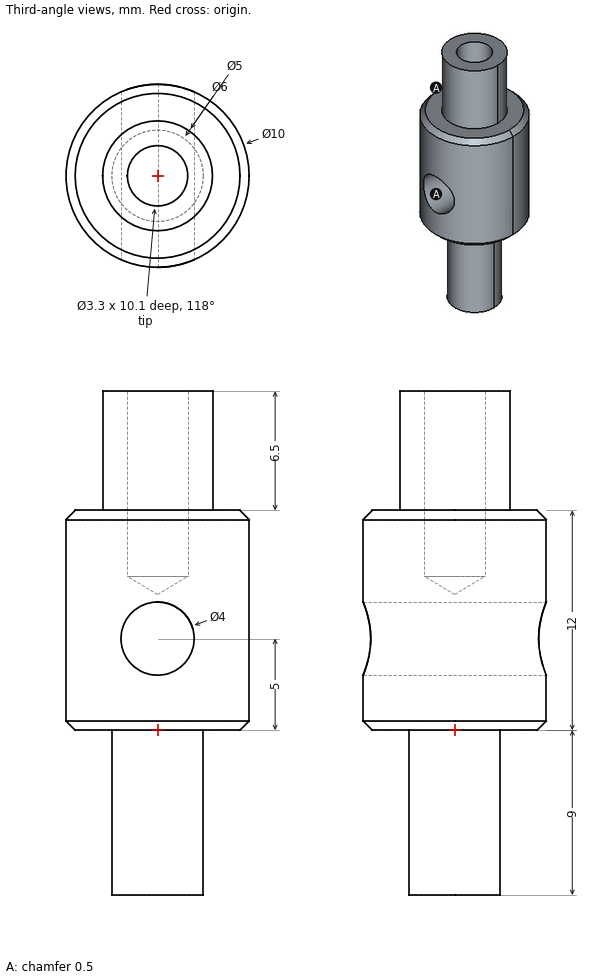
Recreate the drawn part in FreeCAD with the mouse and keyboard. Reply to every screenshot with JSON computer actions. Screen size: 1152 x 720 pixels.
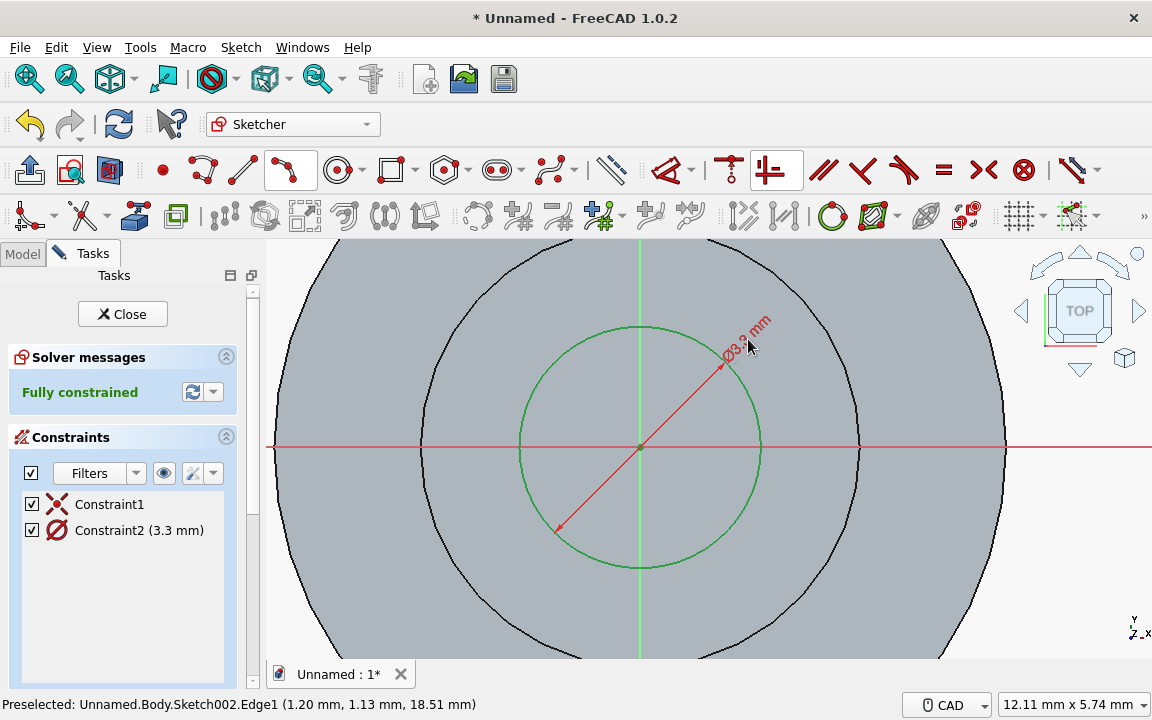
{"action": "left_click", "coordinate": [123, 314]}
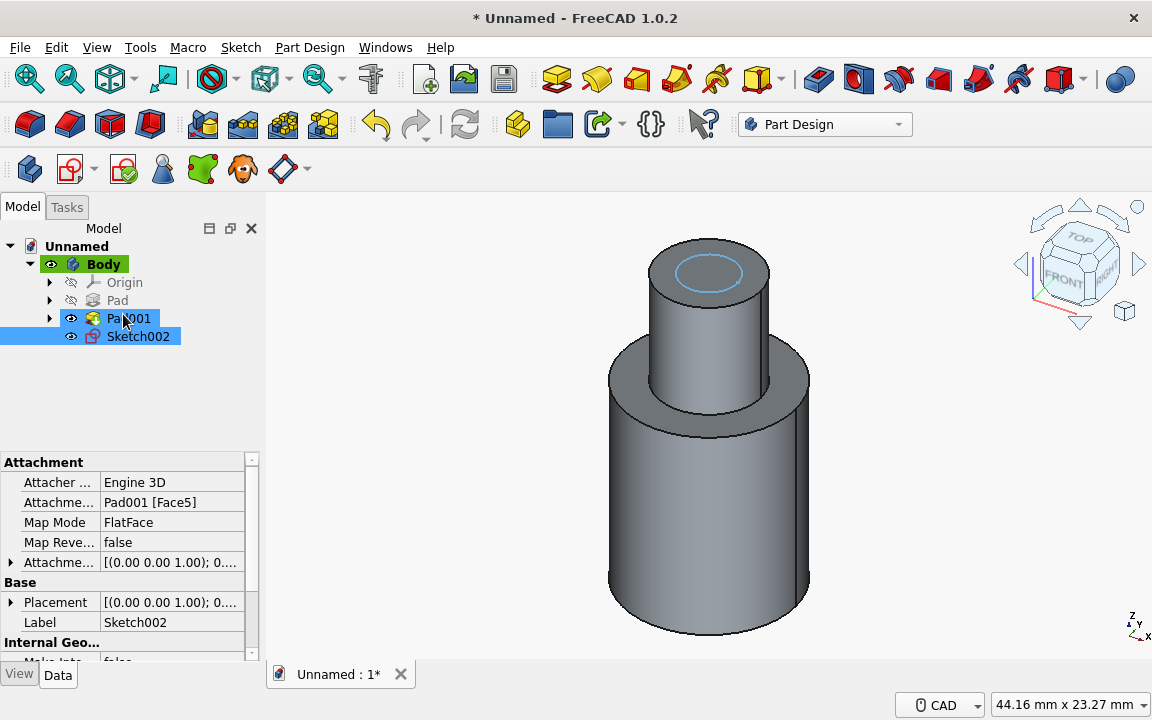
{"action": "left_click", "coordinate": [860, 80]}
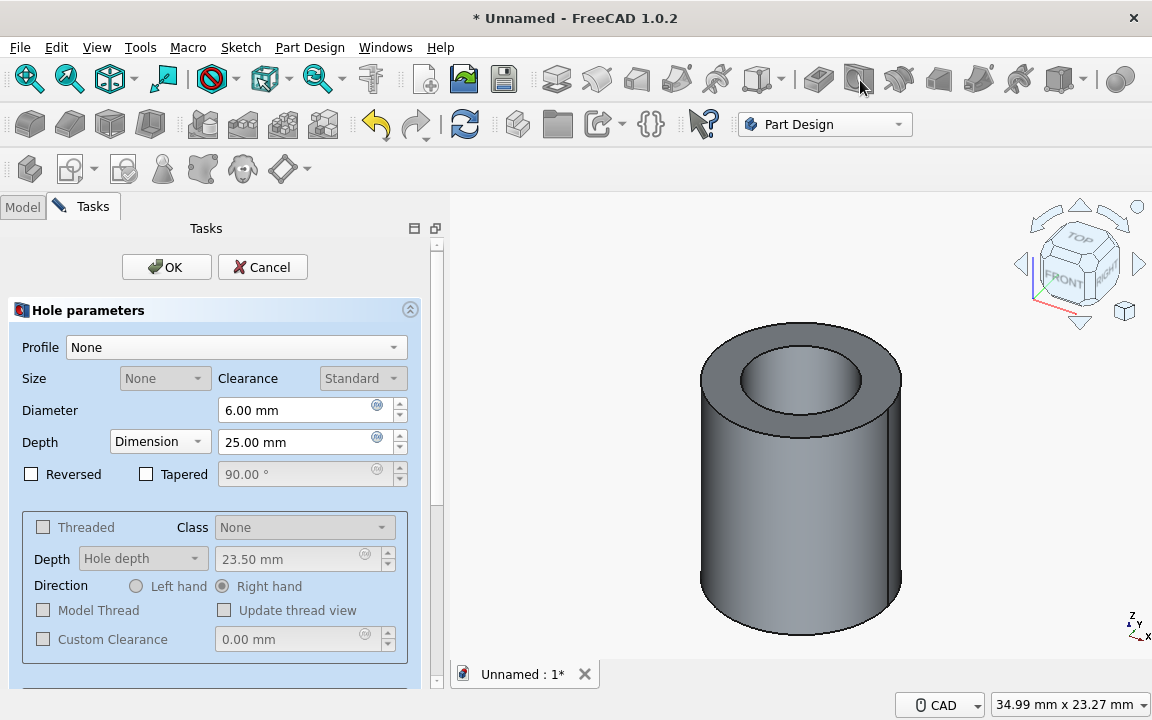
{"action": "triple_click", "coordinate": [305, 410]}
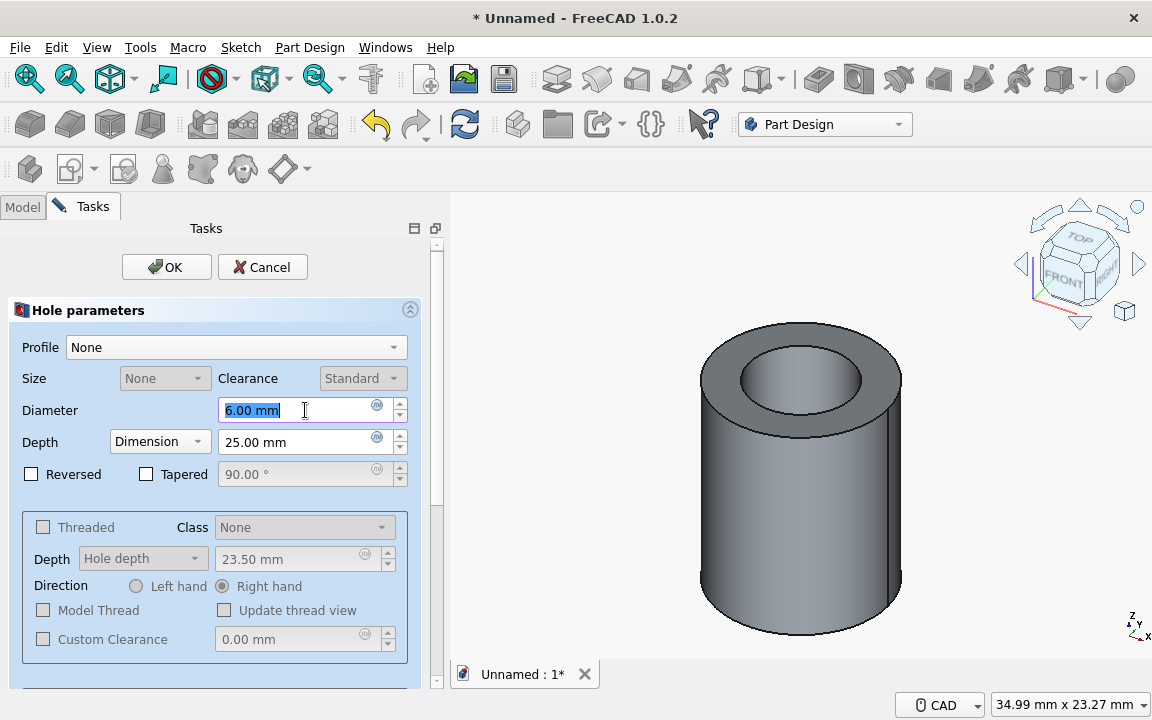
{"action": "type", "text": "3.3"}
{"action": "key", "text": "Tab"}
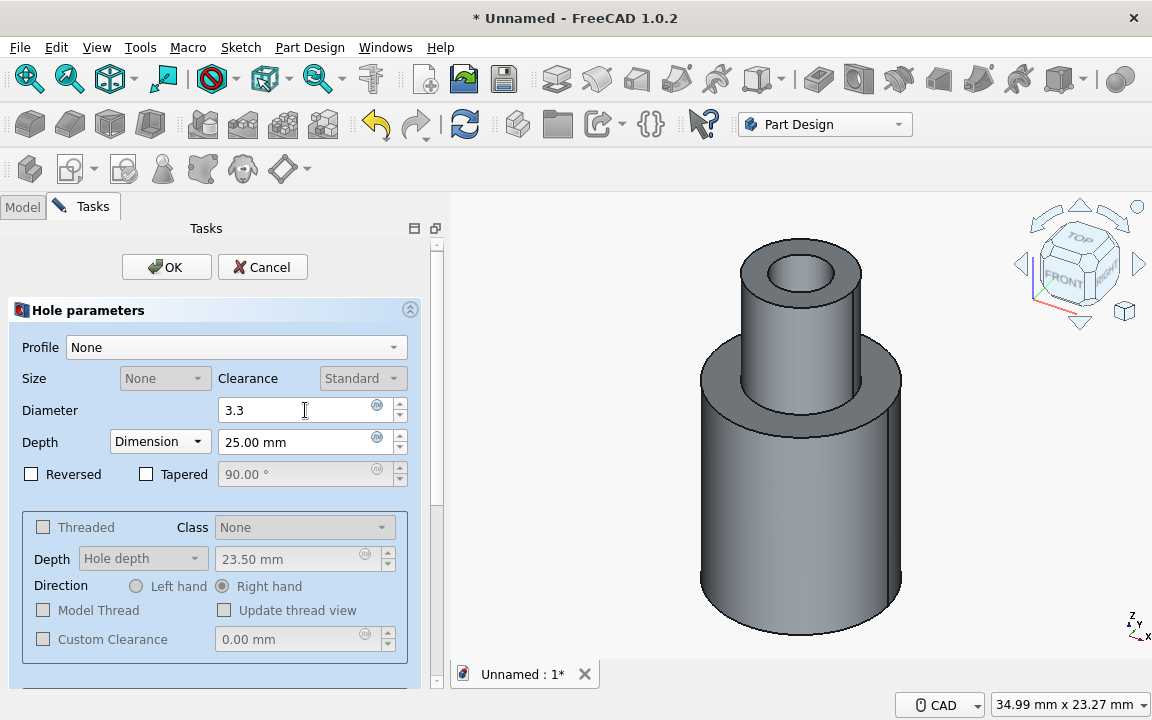
{"action": "triple_click", "coordinate": [305, 442]}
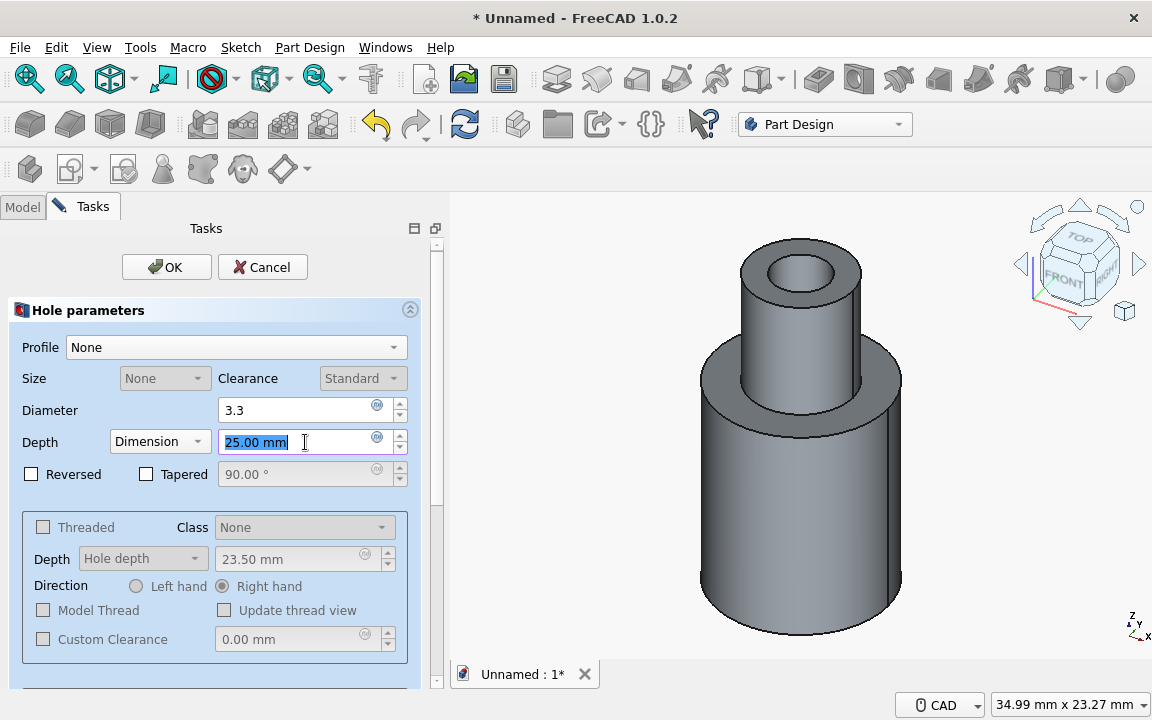
{"action": "type", "text": "10.1"}
{"action": "key", "text": "Tab"}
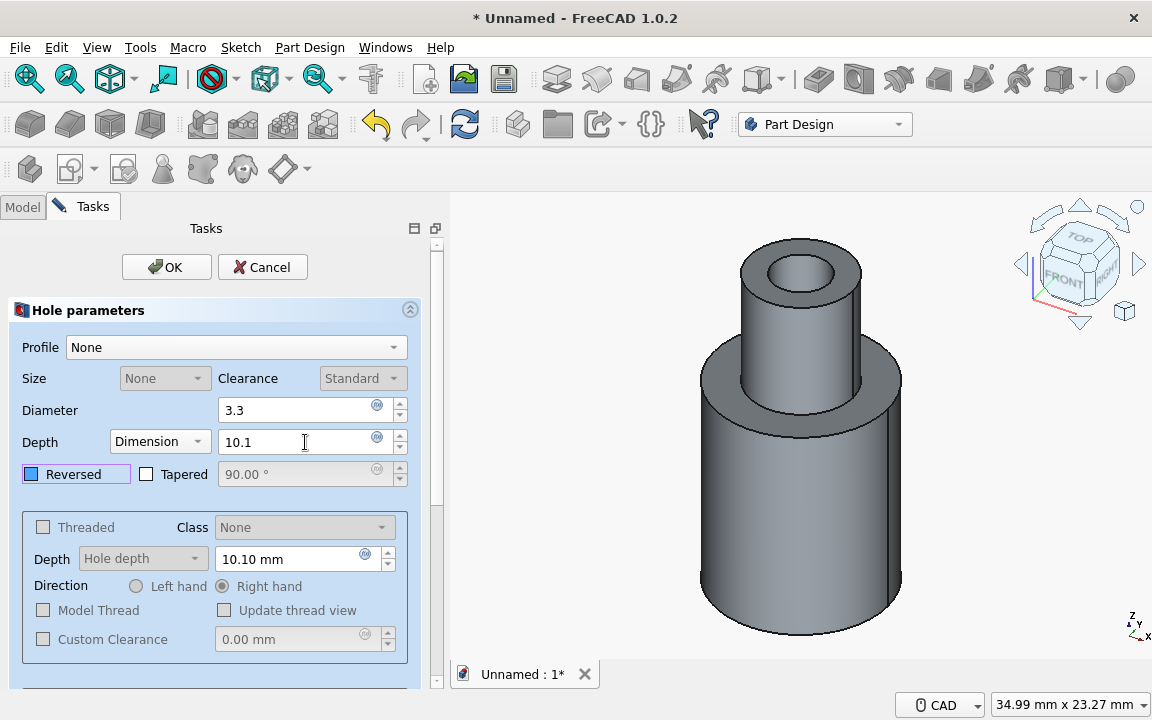
{"action": "left_click", "coordinate": [167, 267]}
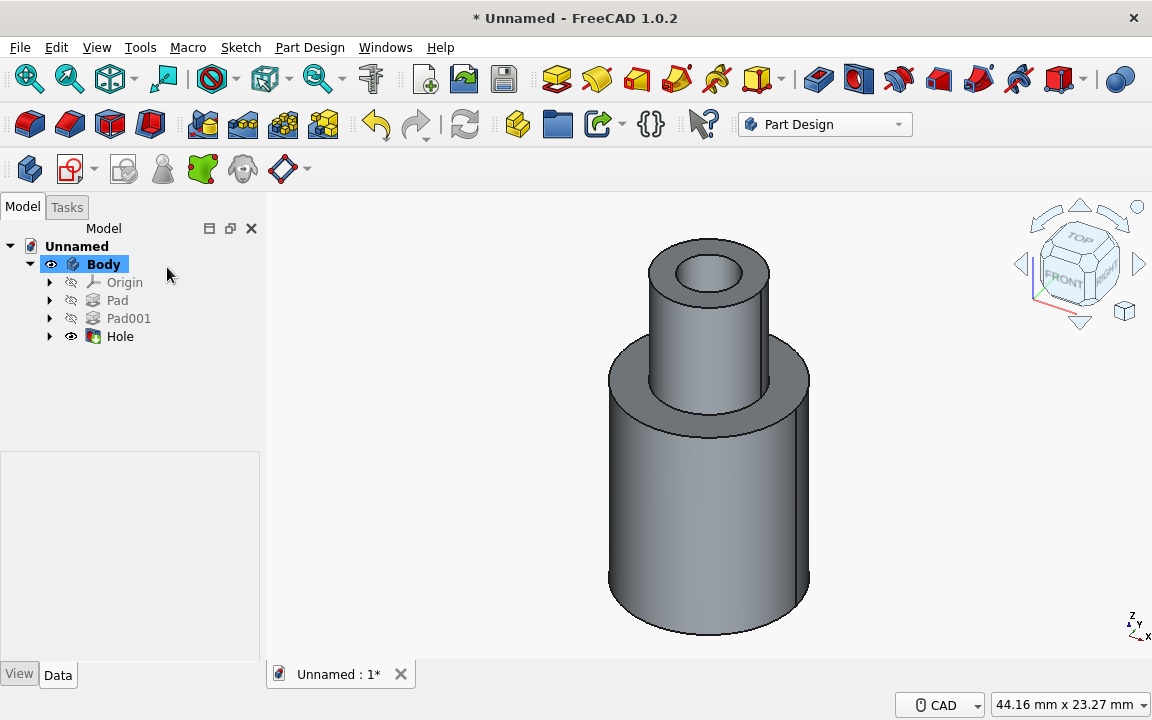
{"action": "left_click", "coordinate": [70, 170]}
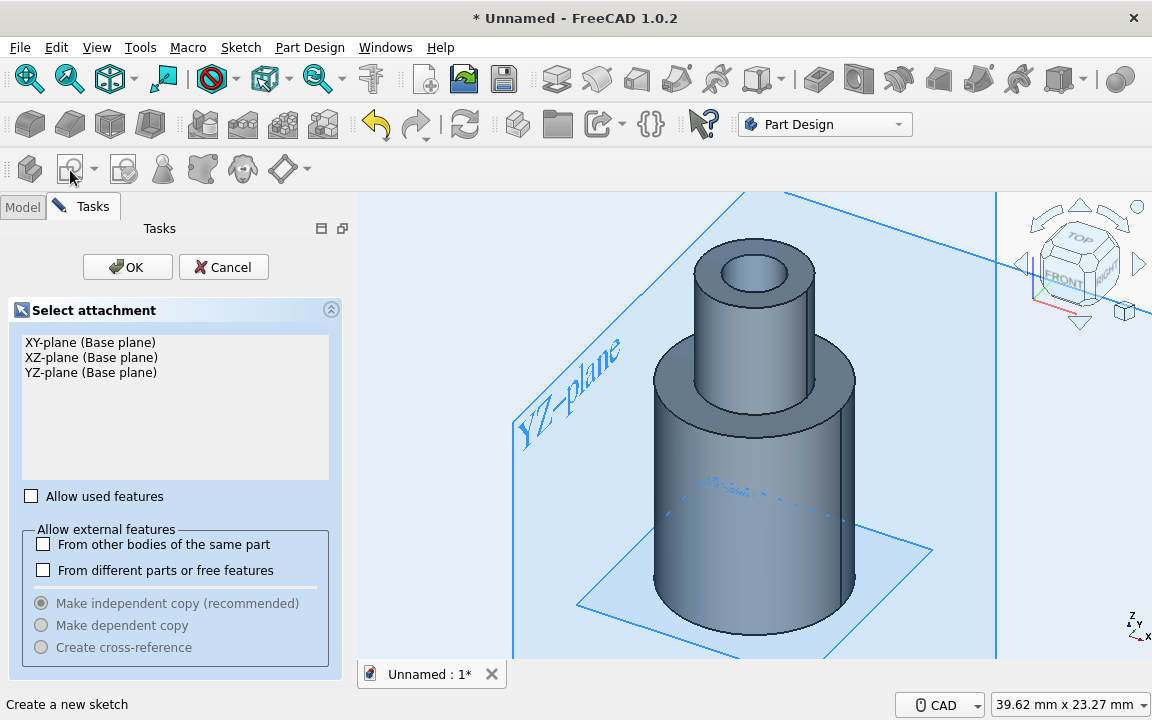
{"action": "left_click", "coordinate": [82, 342]}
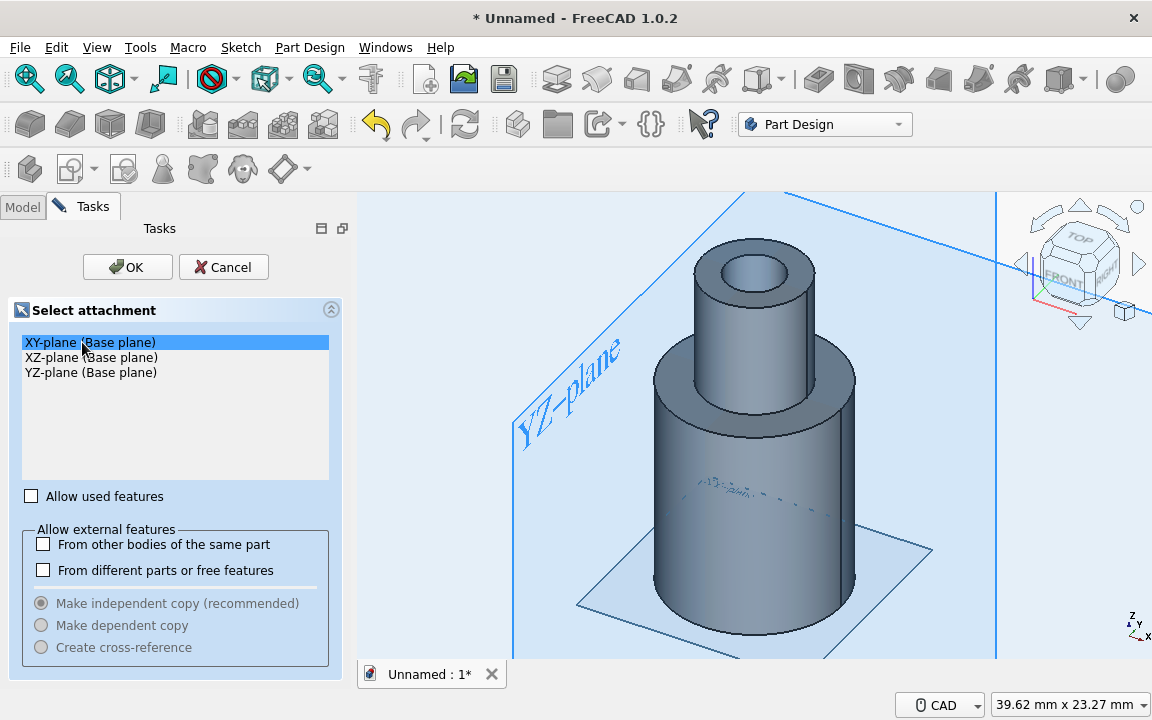
{"action": "left_click", "coordinate": [128, 267]}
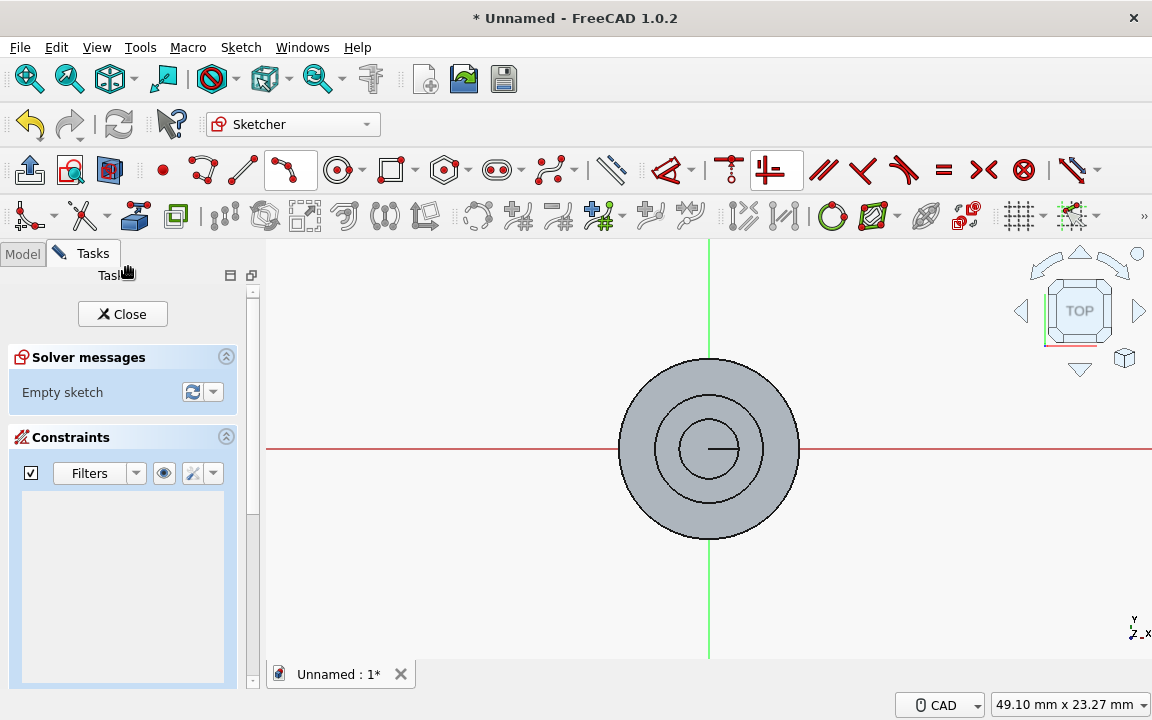
{"action": "key", "text": "q s"}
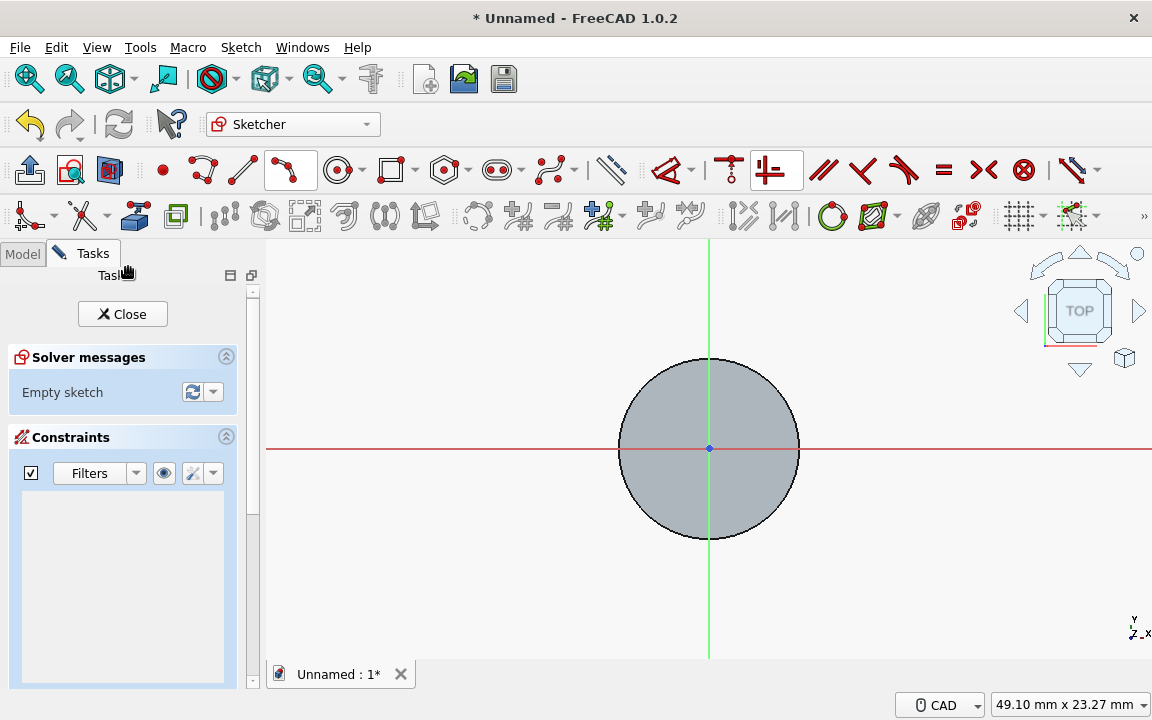
{"action": "scroll", "coordinate": [749, 449], "scroll_direction": "up", "scroll_amount": 5}